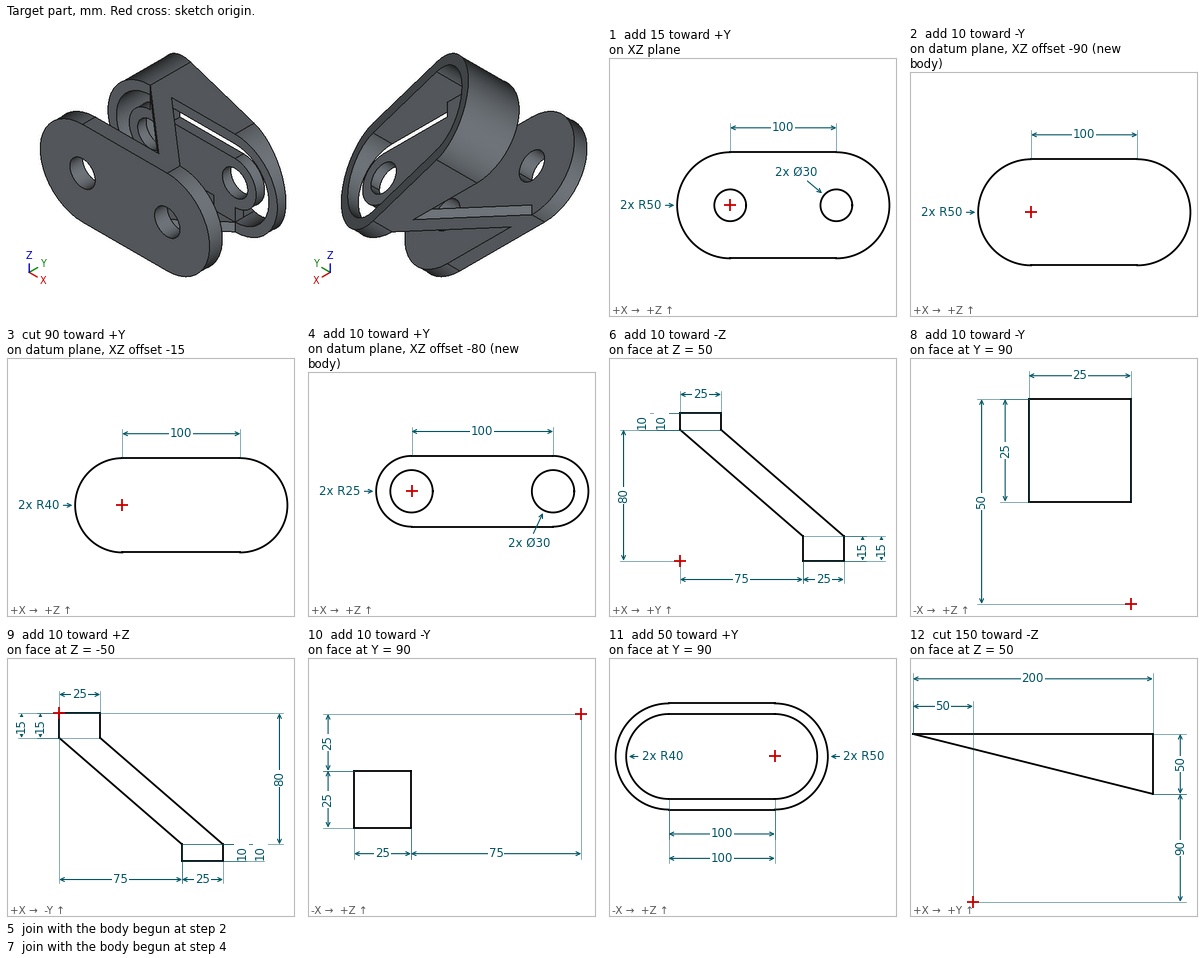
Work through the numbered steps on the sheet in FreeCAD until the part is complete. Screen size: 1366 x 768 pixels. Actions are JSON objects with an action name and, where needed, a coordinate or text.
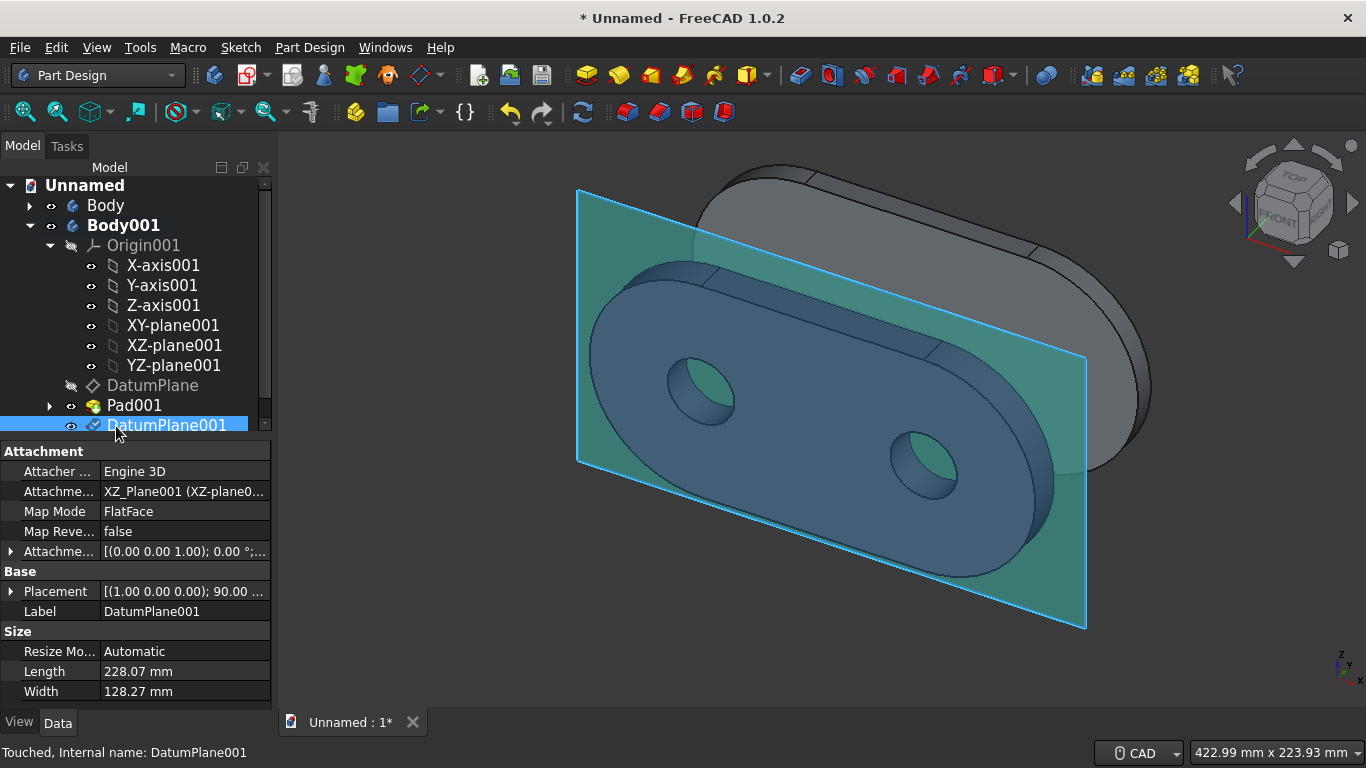
{"action": "left_click", "coordinate": [248, 76]}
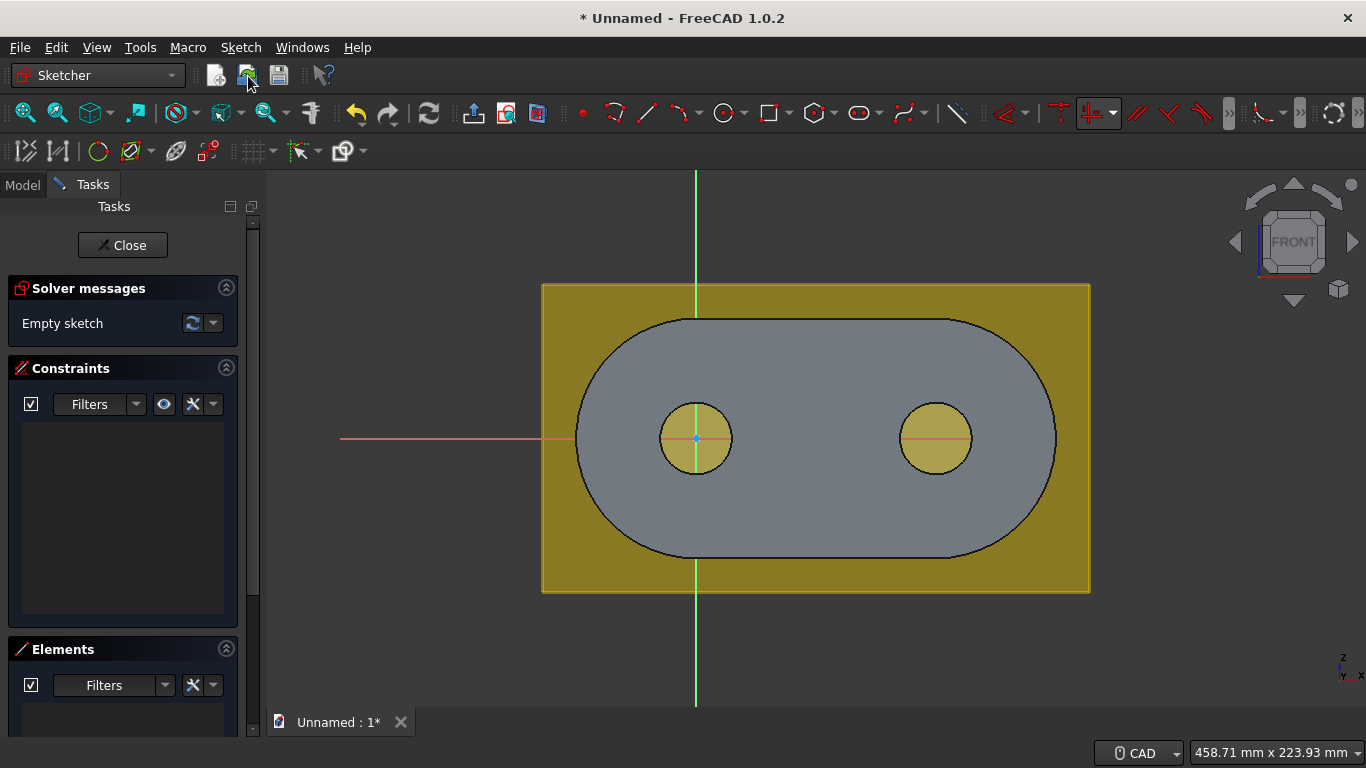
{"action": "scroll", "coordinate": [955, 439], "scroll_direction": "up", "scroll_amount": 2}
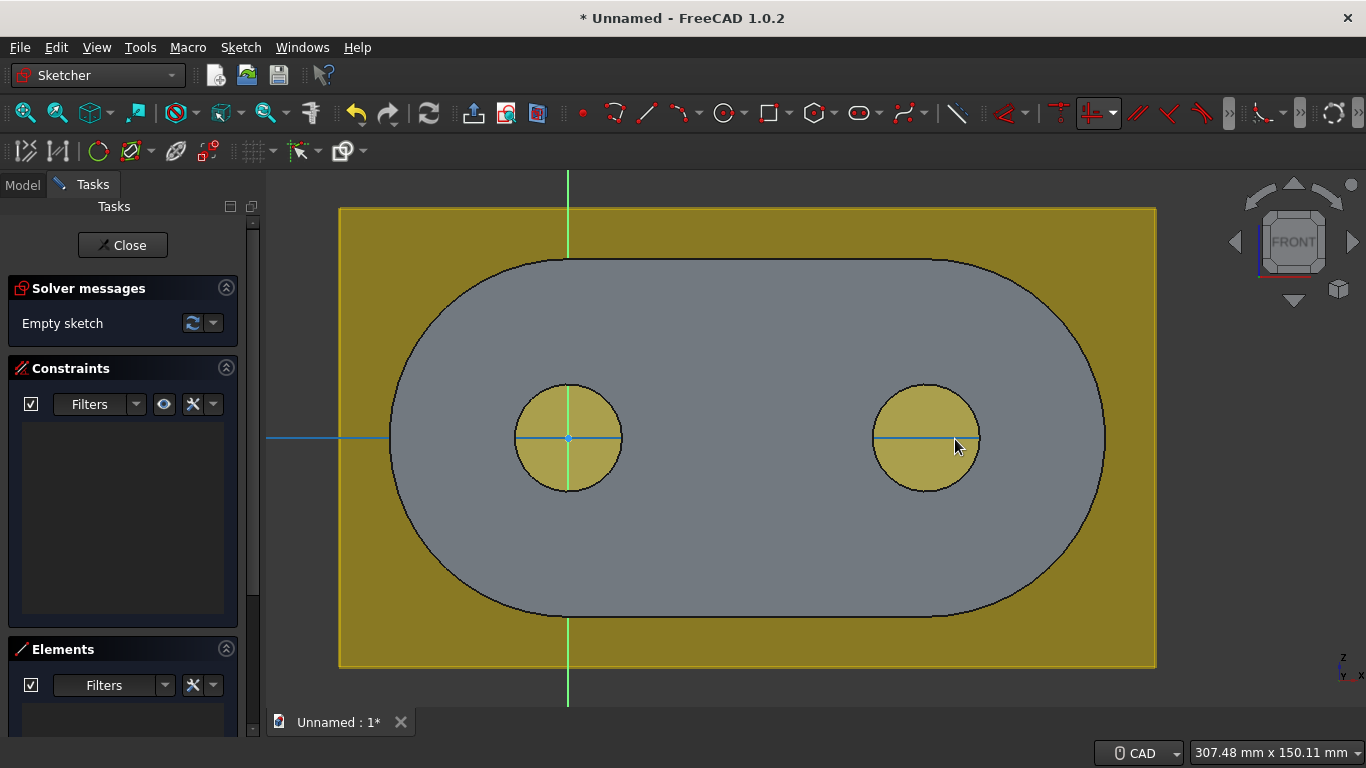
{"action": "left_click", "coordinate": [860, 114]}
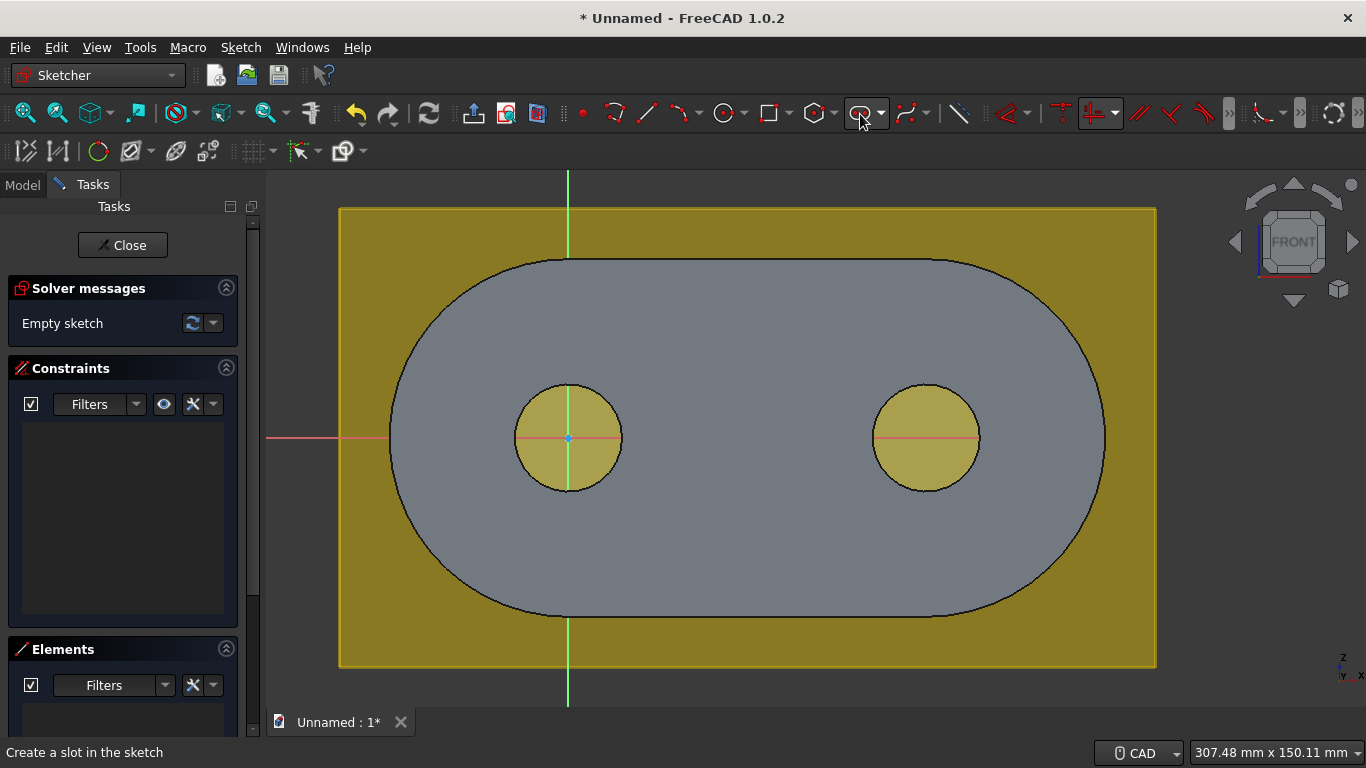
{"action": "left_click", "coordinate": [568, 438]}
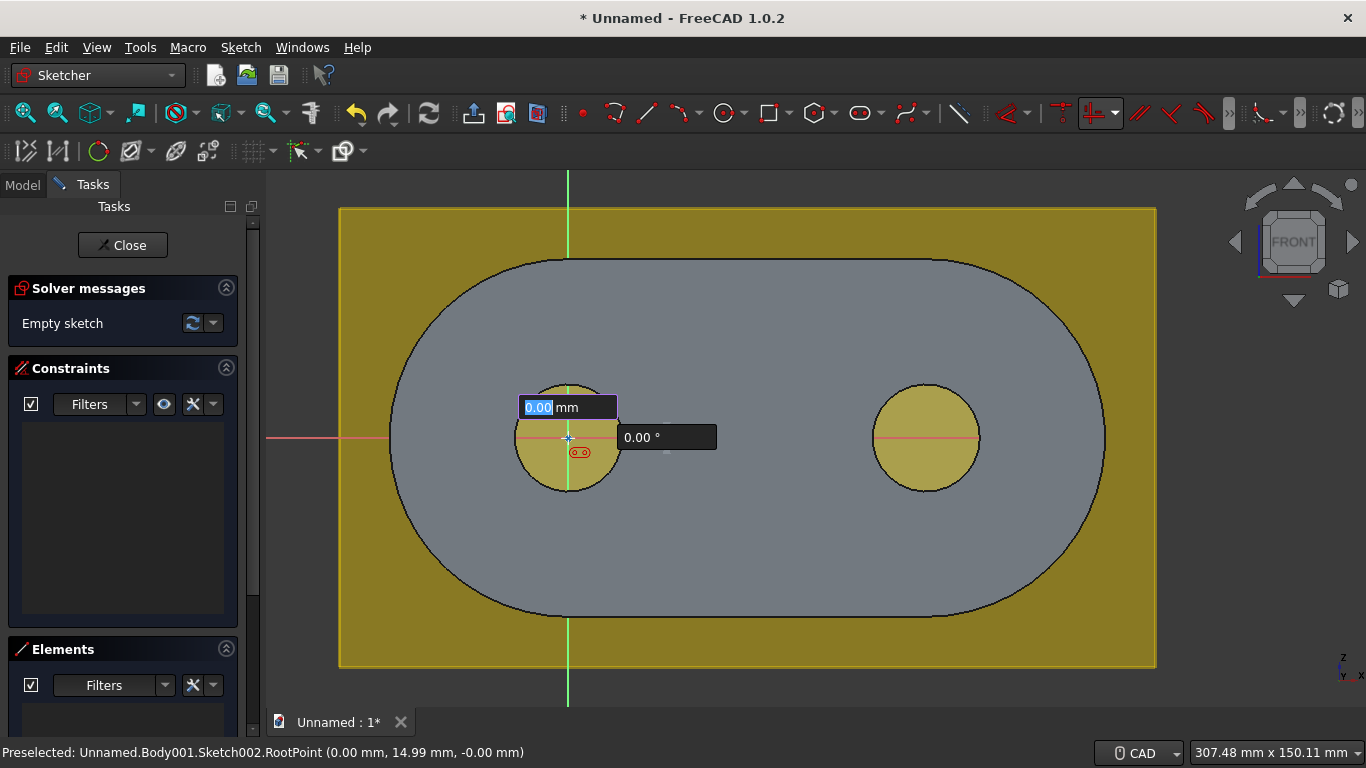
{"action": "left_click", "coordinate": [926, 429]}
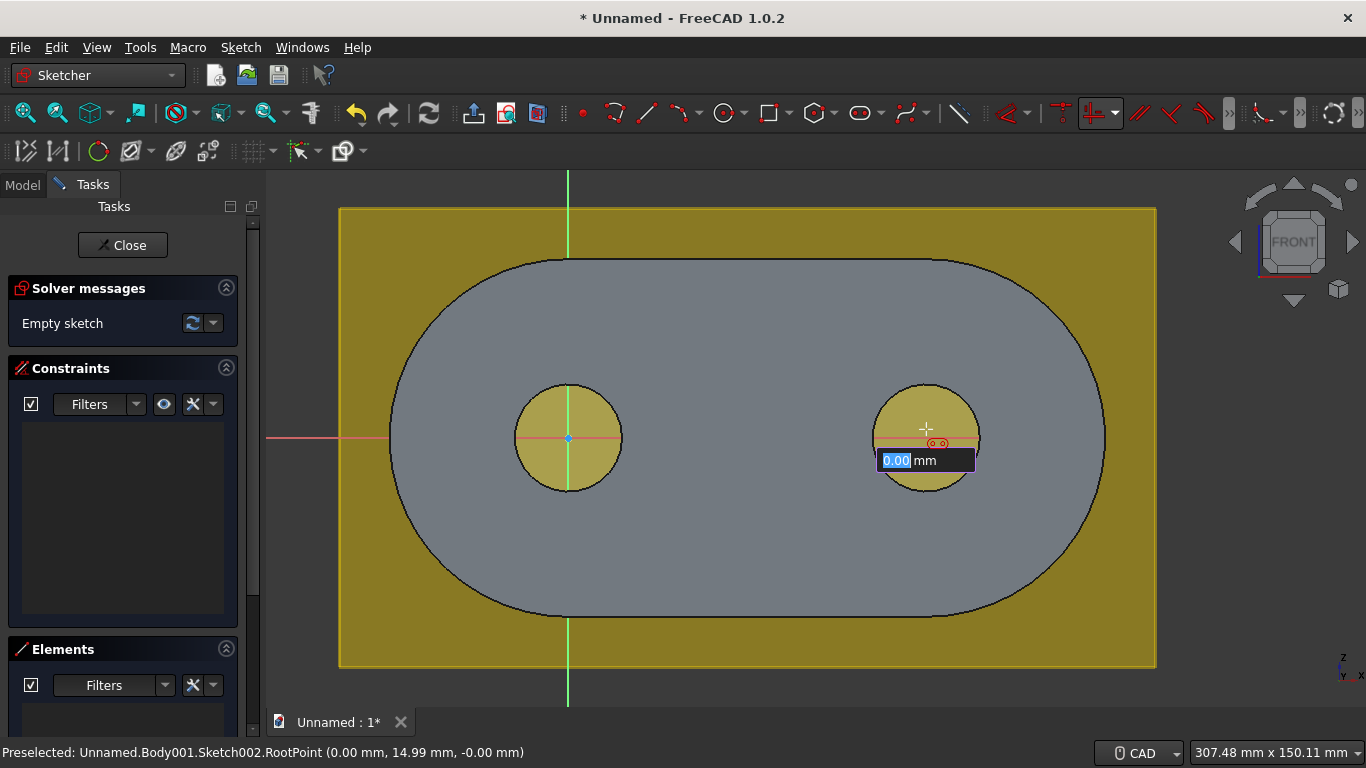
{"action": "left_click", "coordinate": [747, 581]}
{"action": "key", "text": "Escape"}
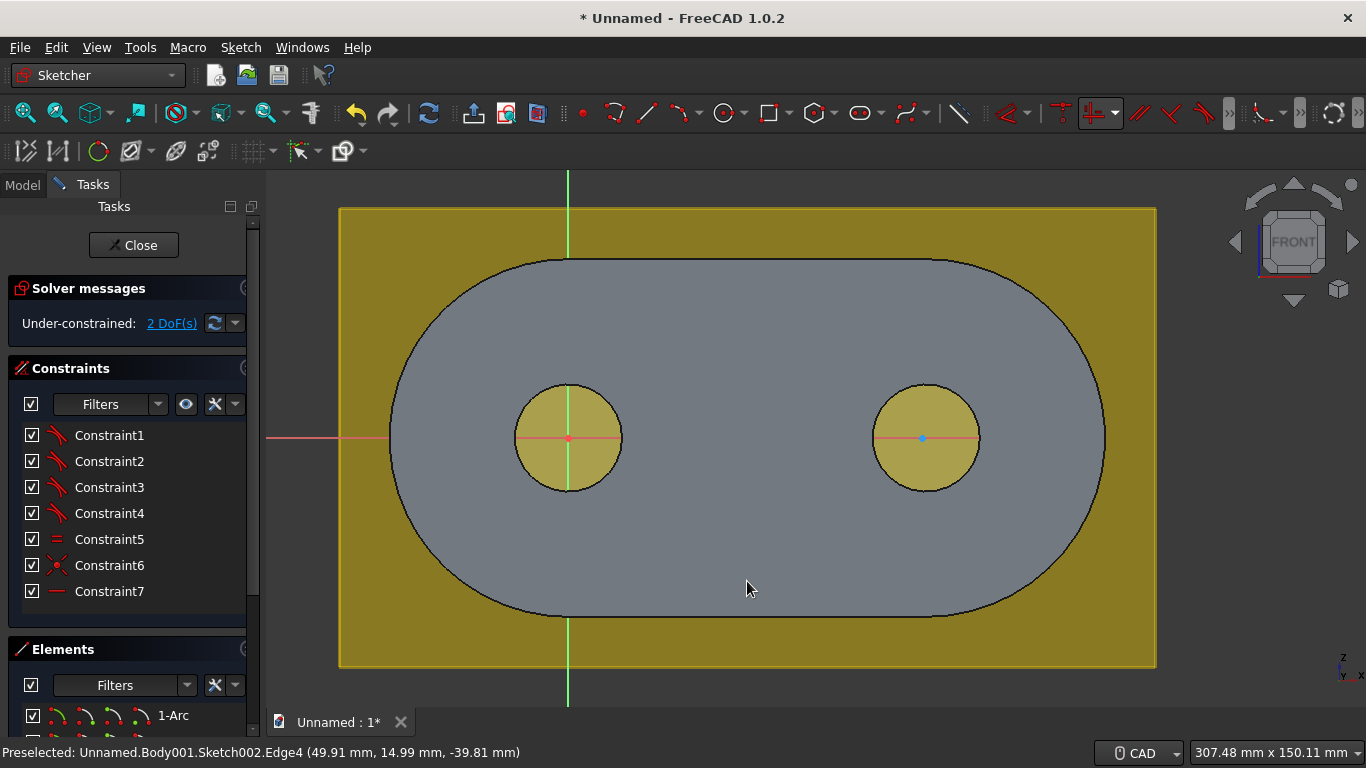
{"action": "left_click", "coordinate": [1006, 114]}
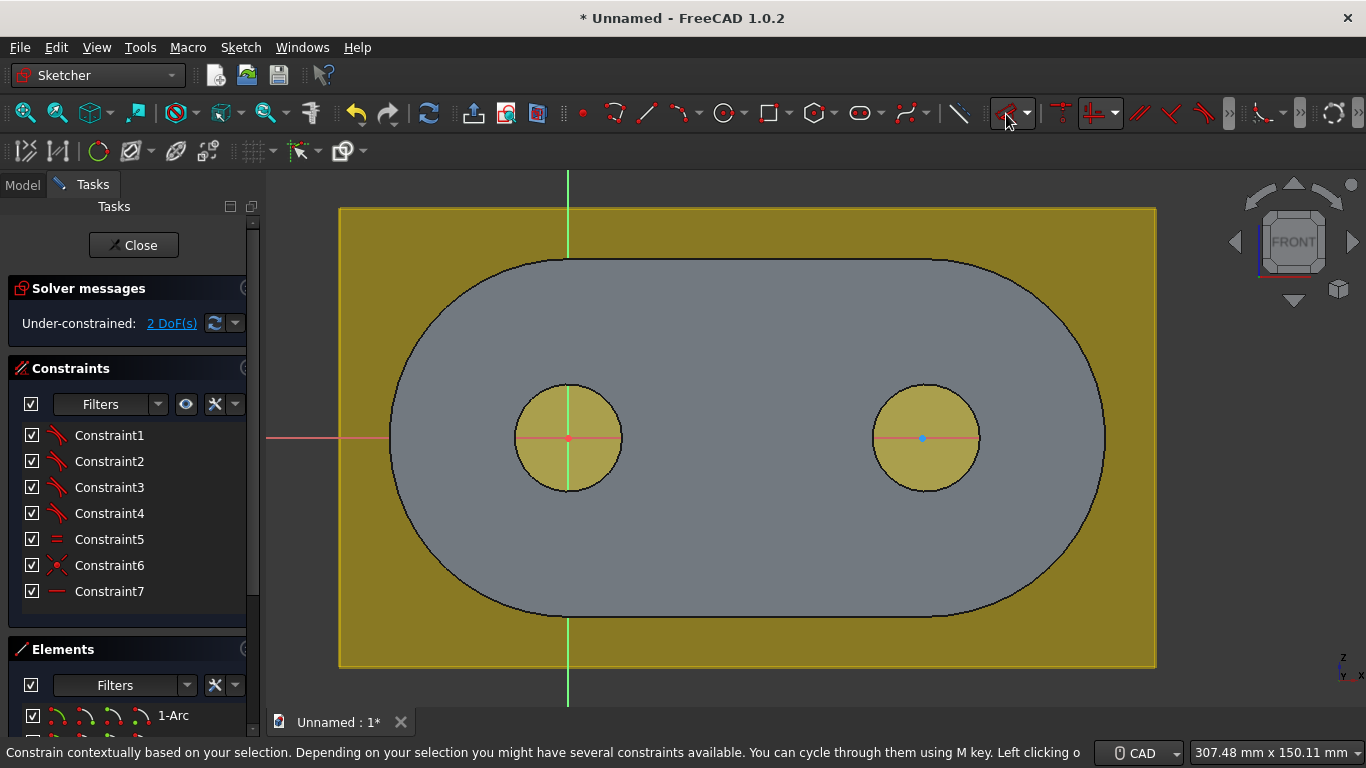
{"action": "left_click", "coordinate": [453, 354]}
{"action": "left_click", "coordinate": [427, 335]}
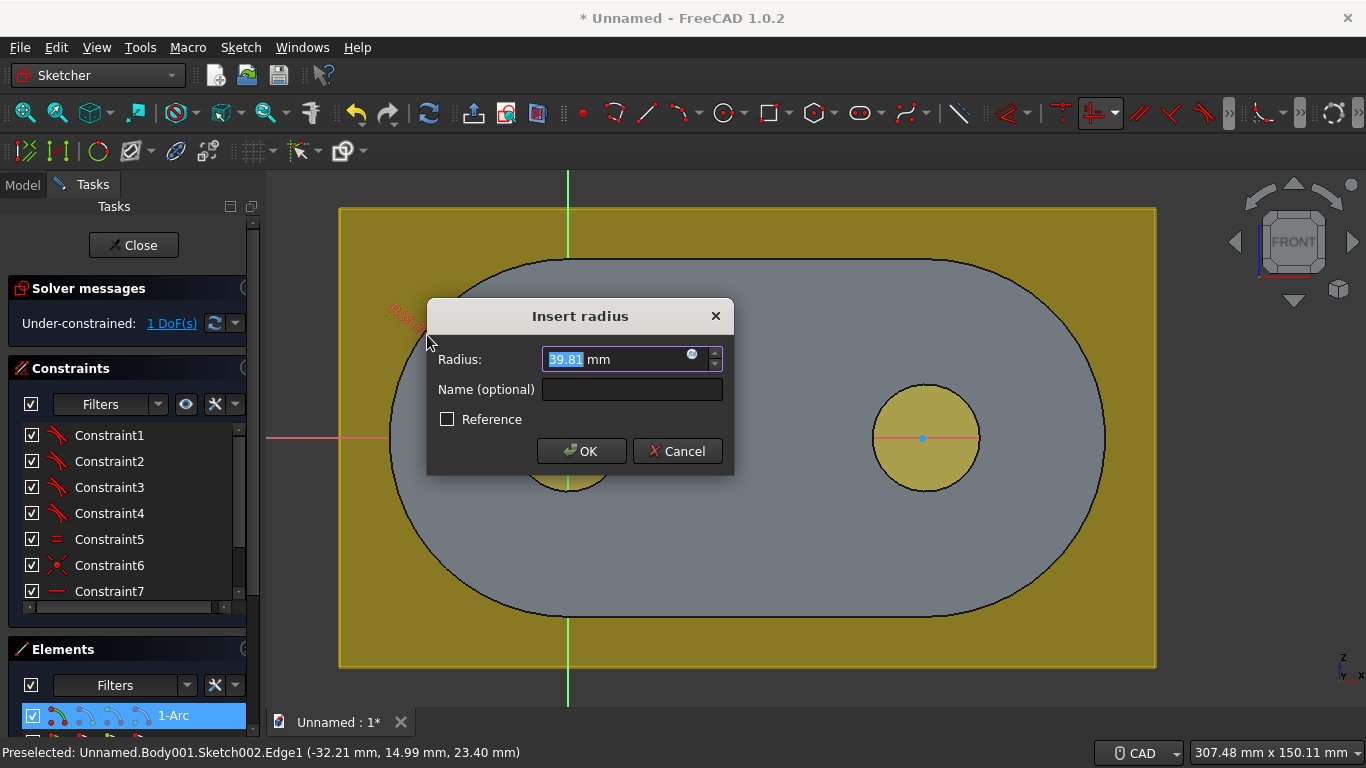
{"action": "type", "text": "40"}
{"action": "key", "text": "Return"}